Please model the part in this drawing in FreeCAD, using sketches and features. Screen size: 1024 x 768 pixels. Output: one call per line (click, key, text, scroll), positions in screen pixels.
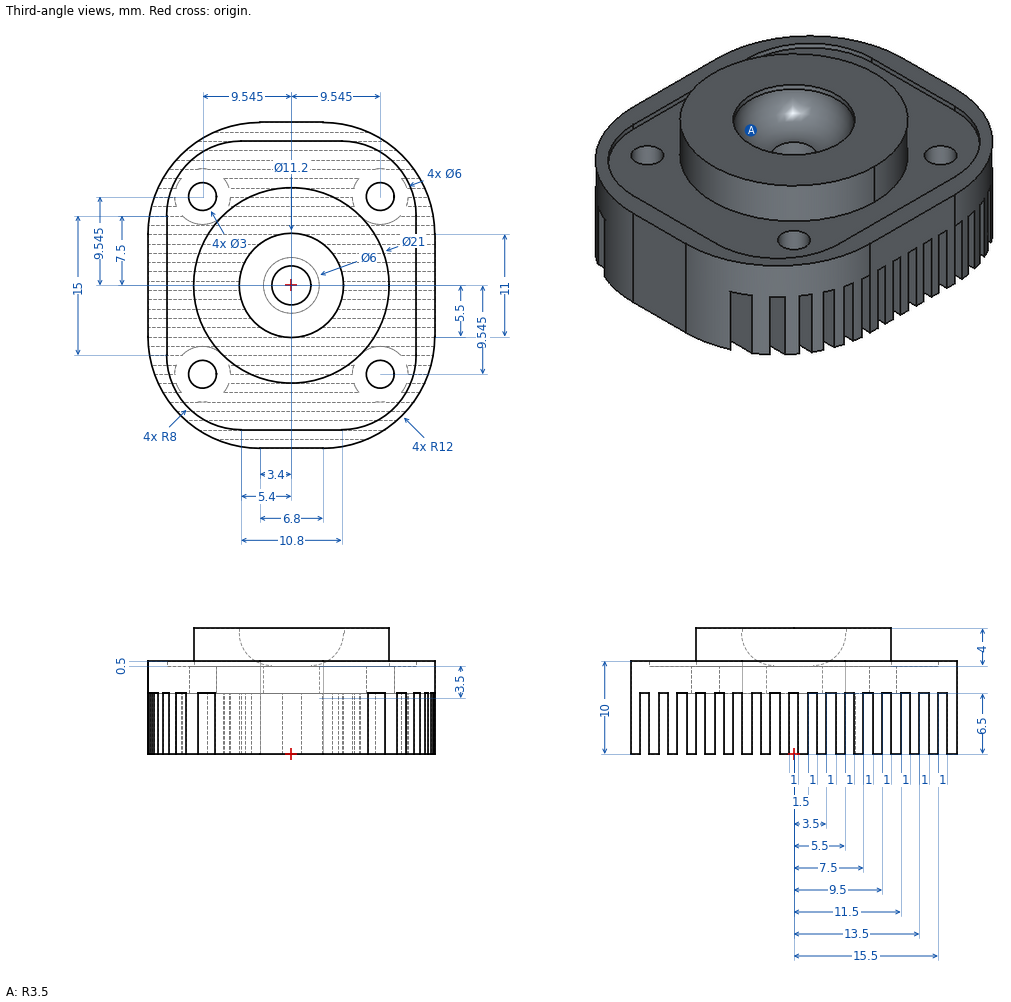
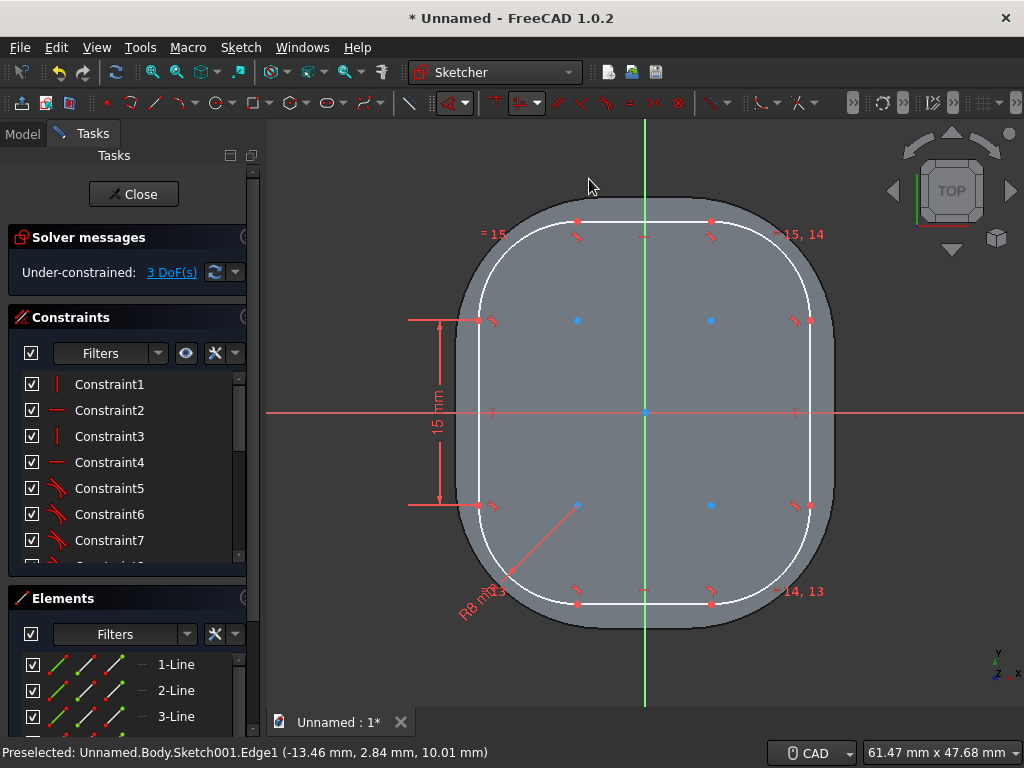
click(618, 604)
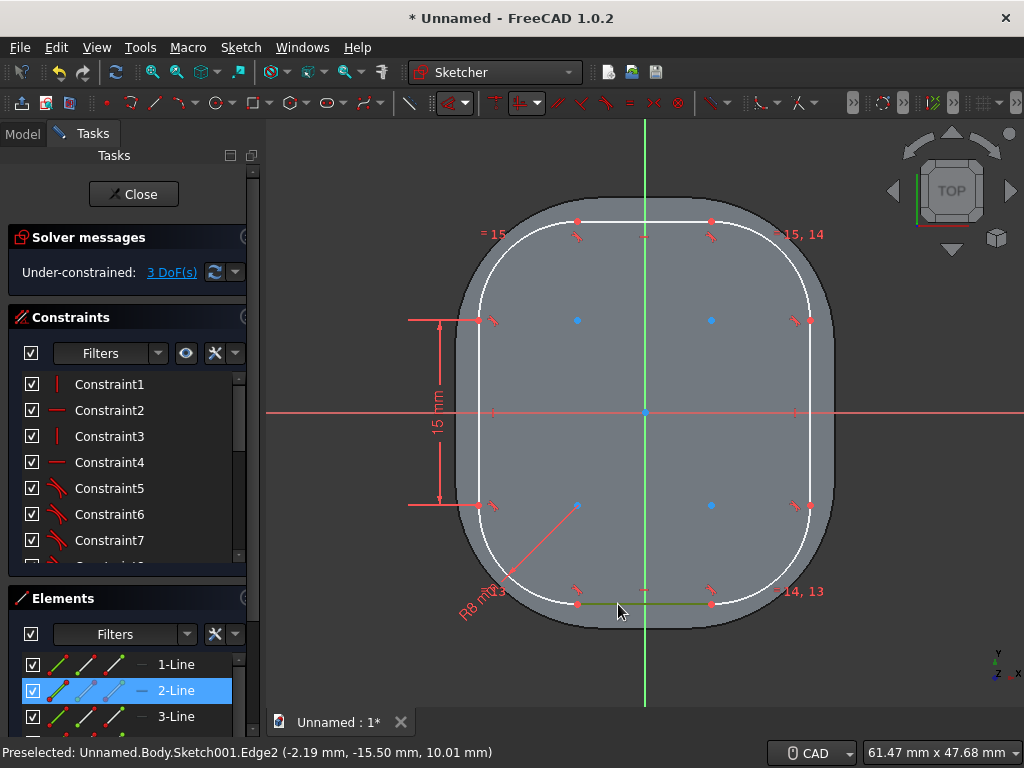
key(l)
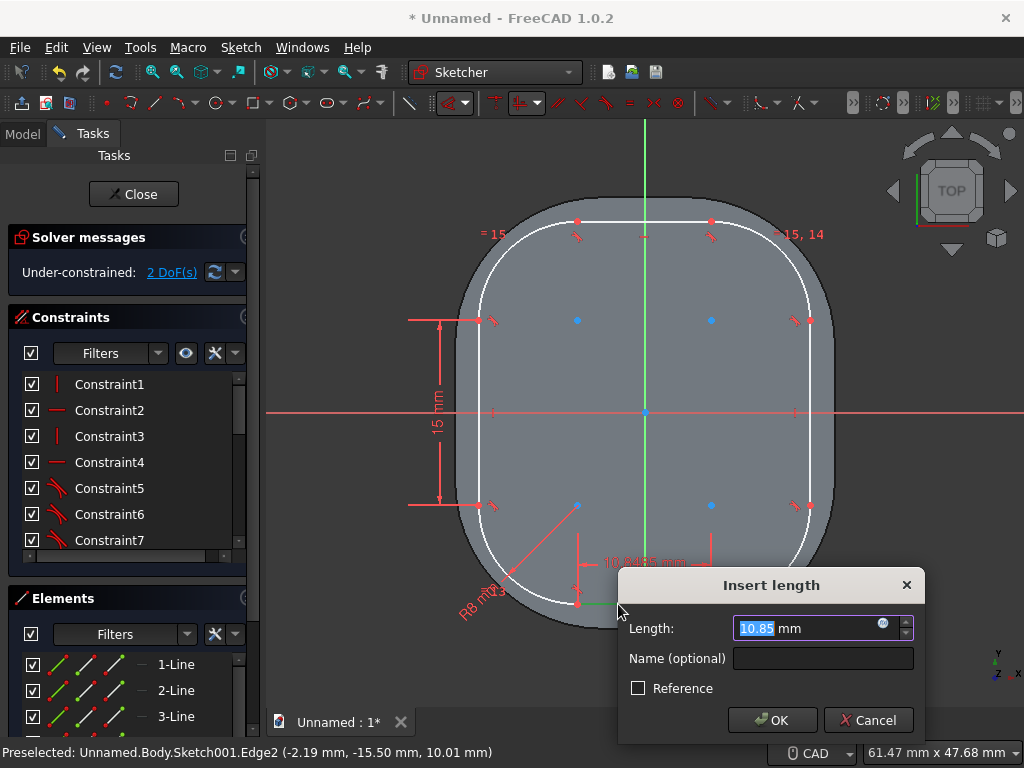
text(10.8)
key(Return)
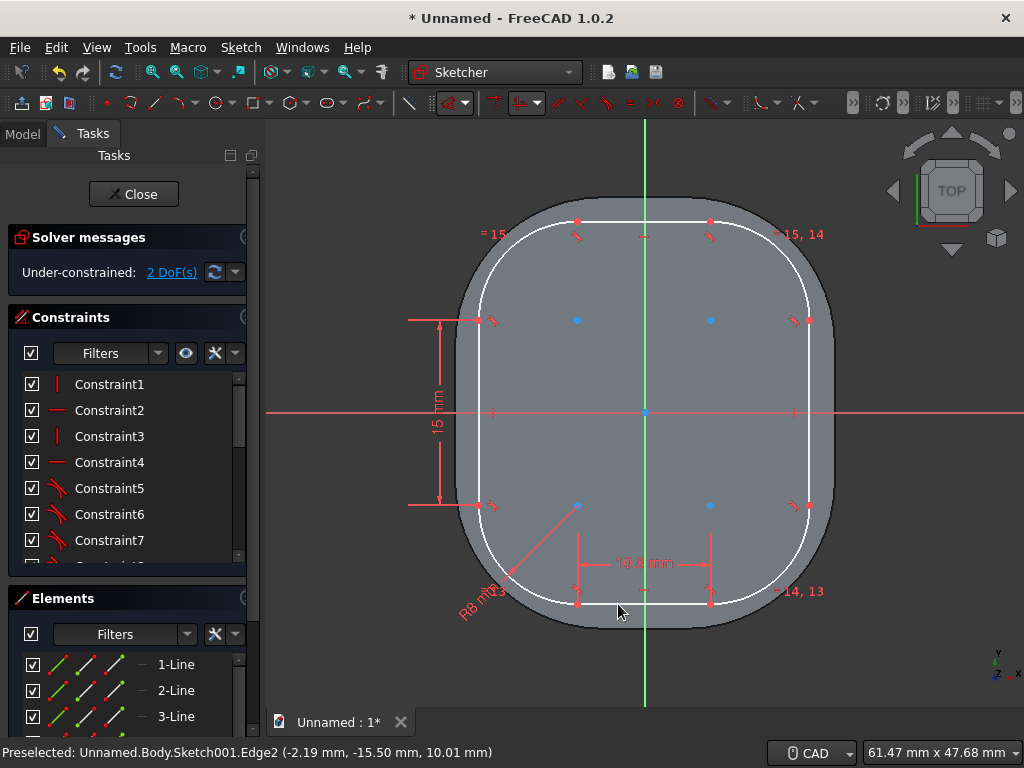
click(479, 320)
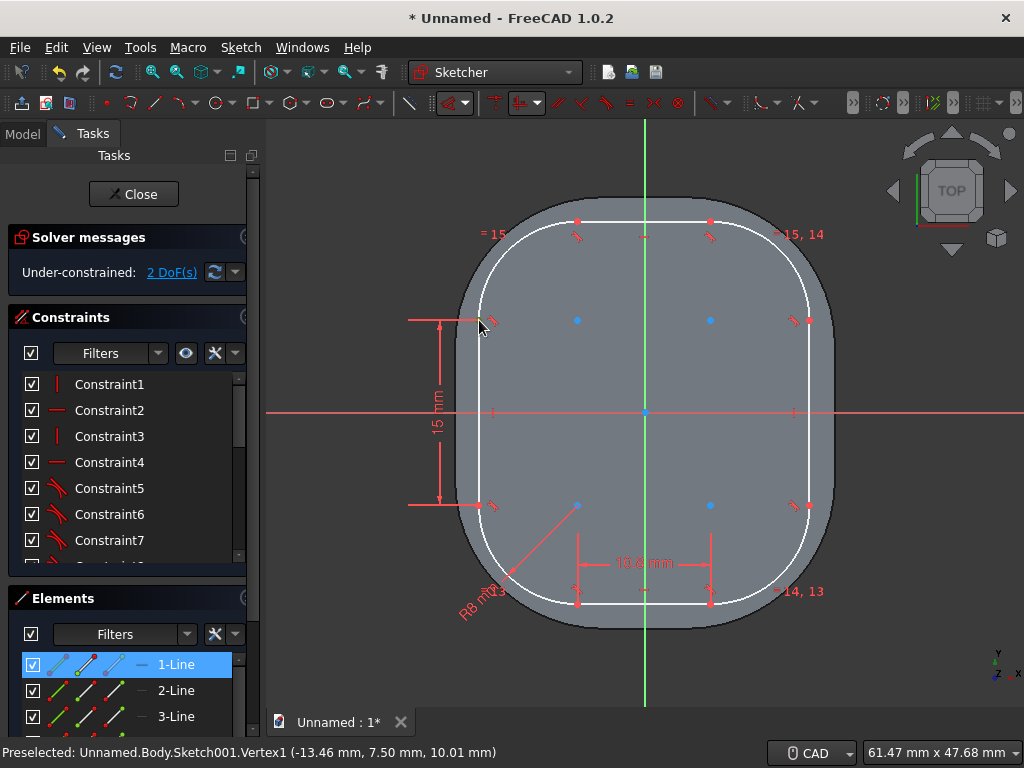
click(468, 104)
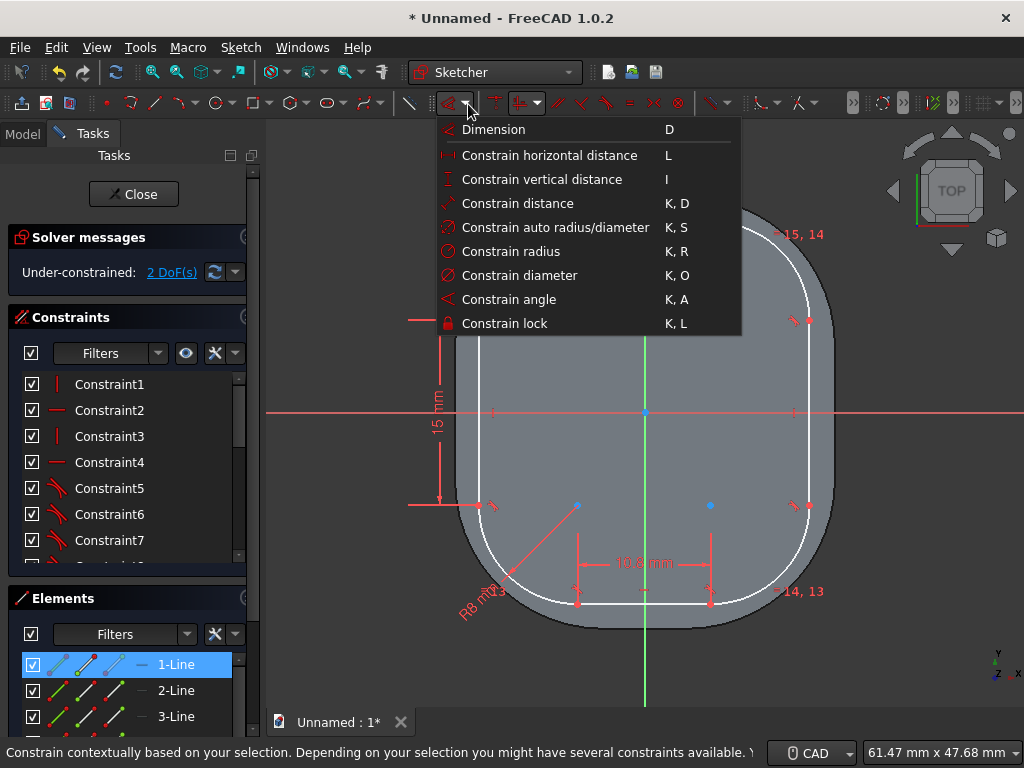
click(589, 179)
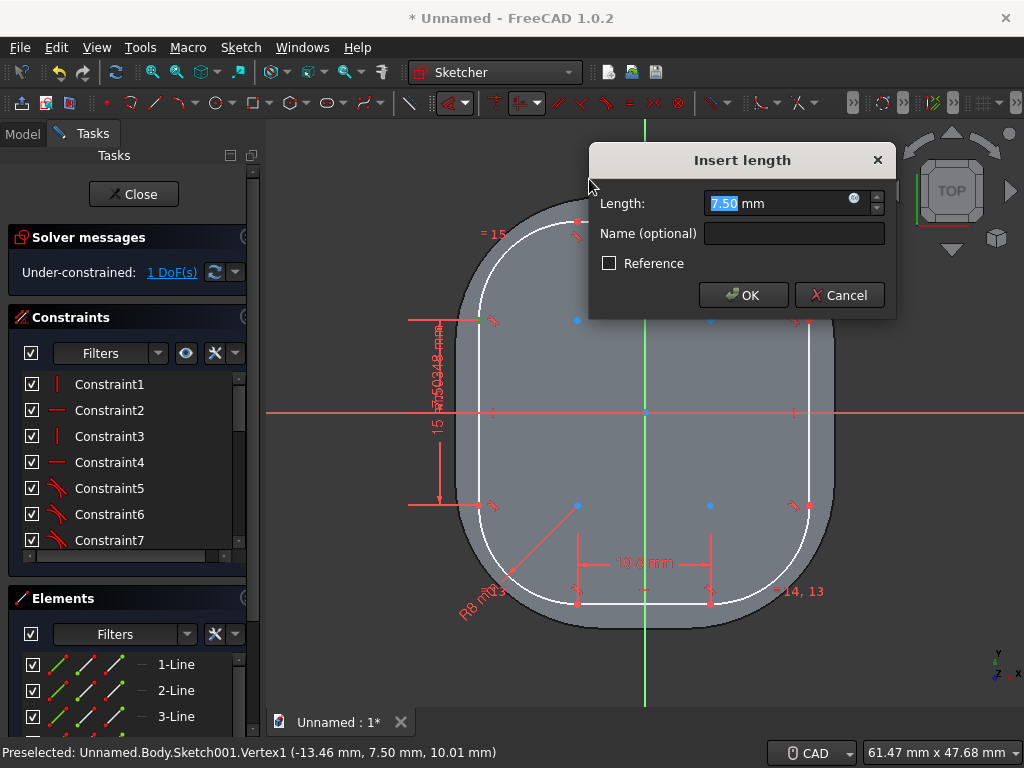
text(7.5)
key(Return)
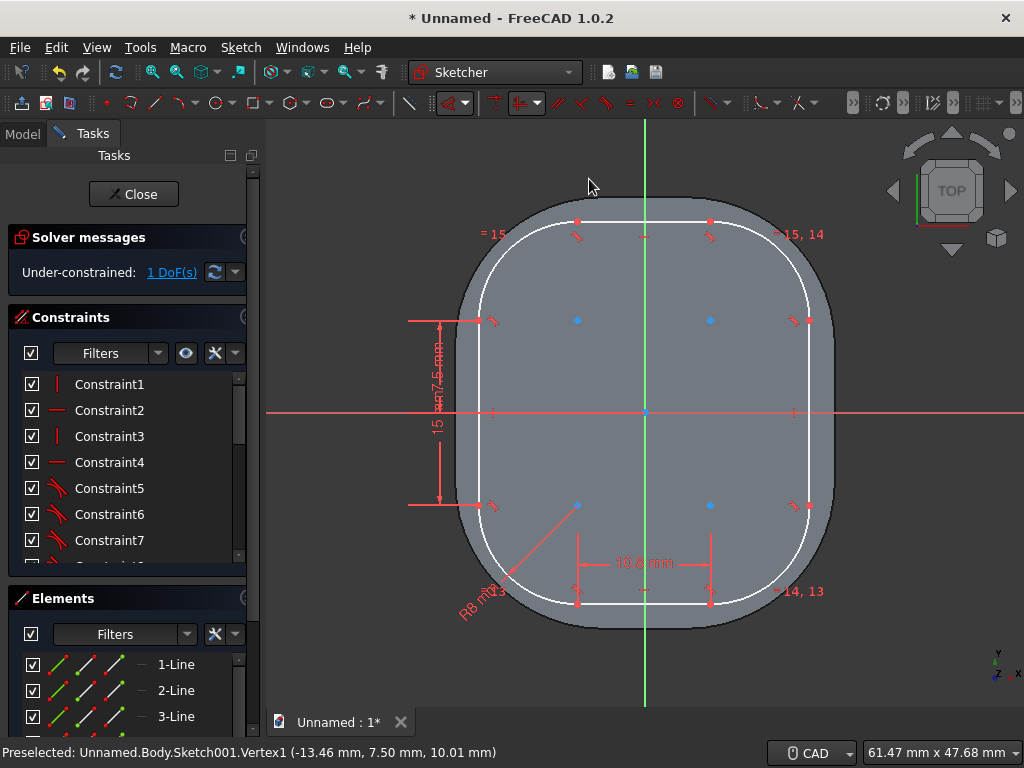
click(578, 604)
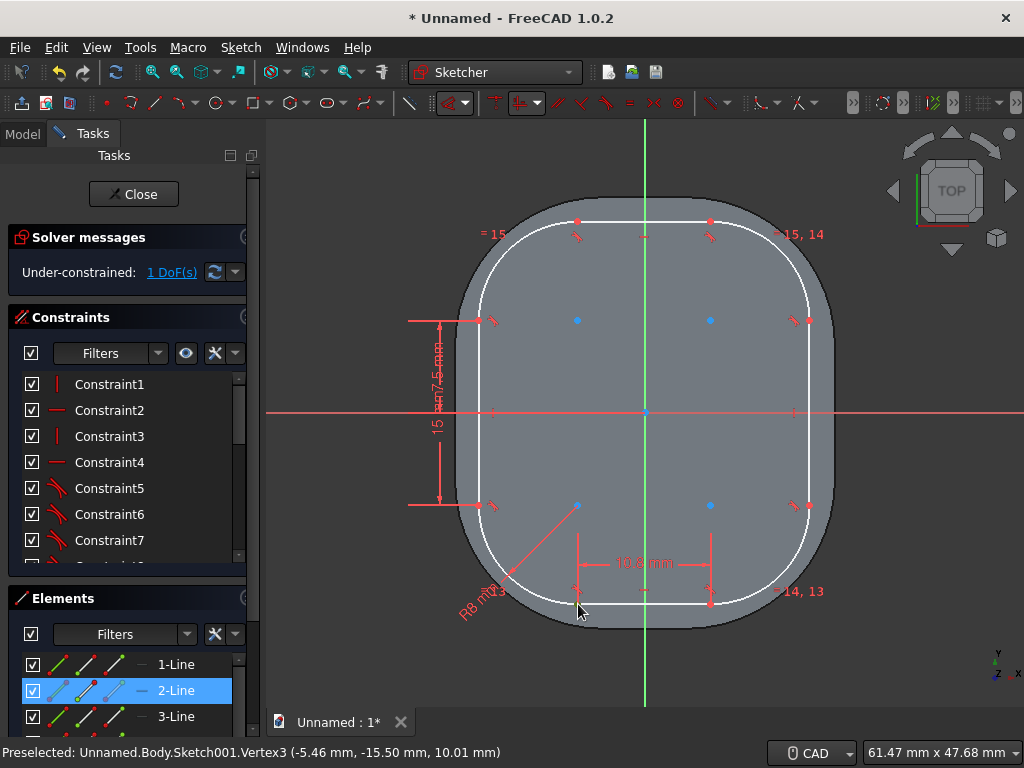
key(l)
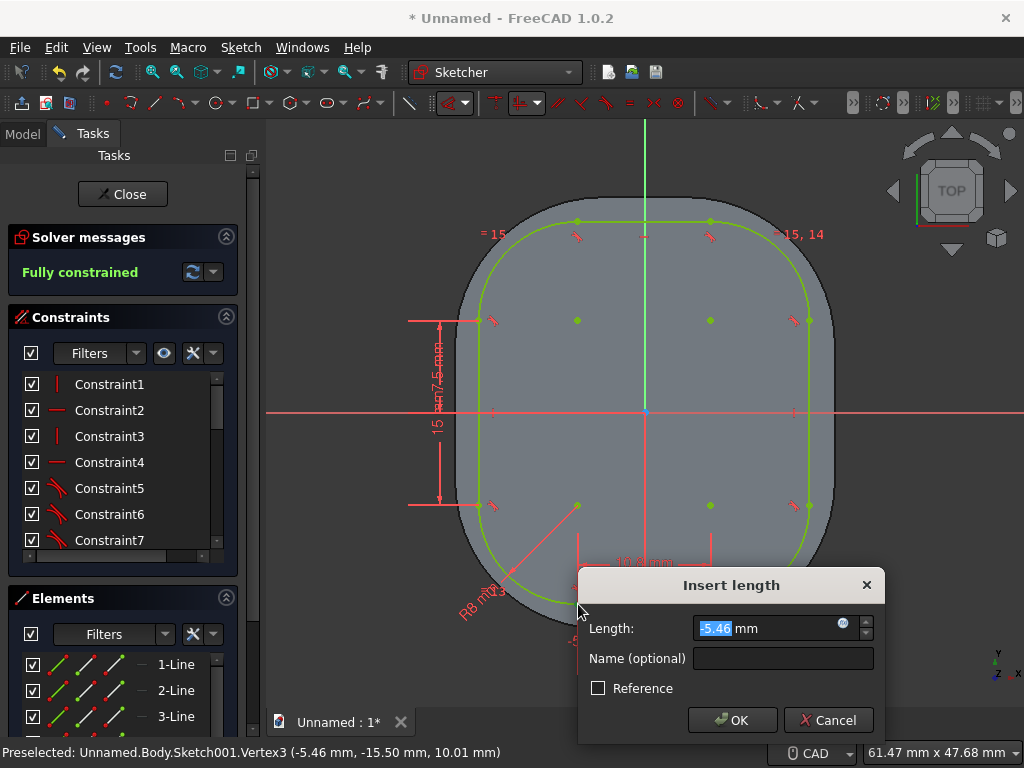
text(-5.4)
key(Return)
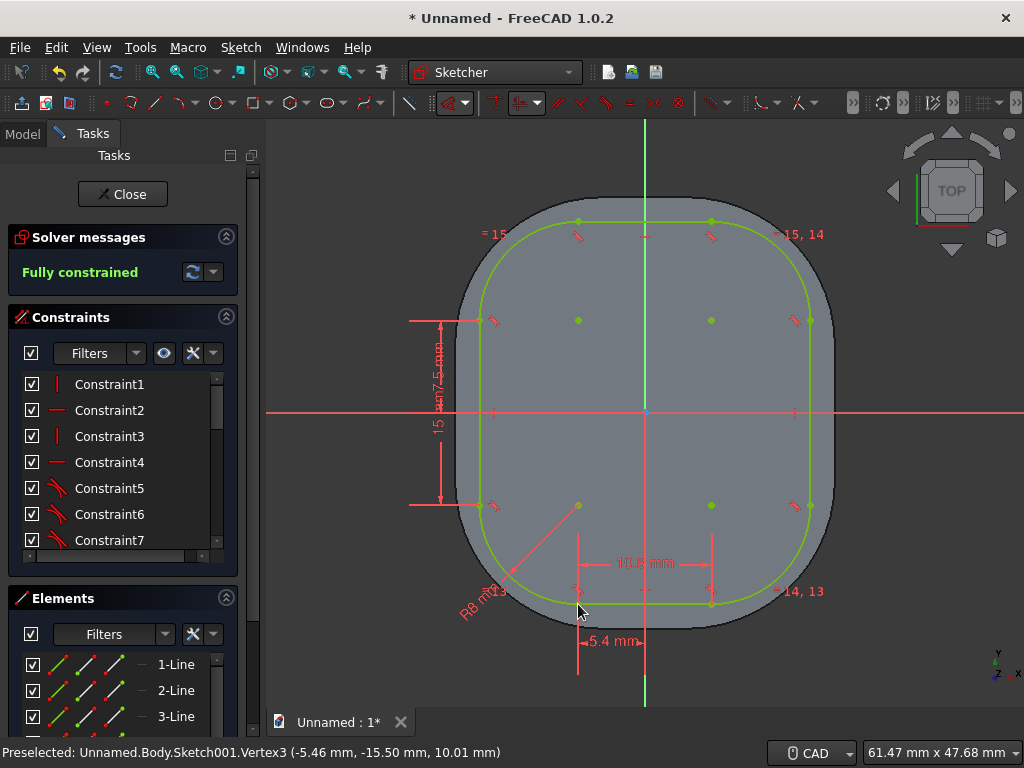
click(123, 194)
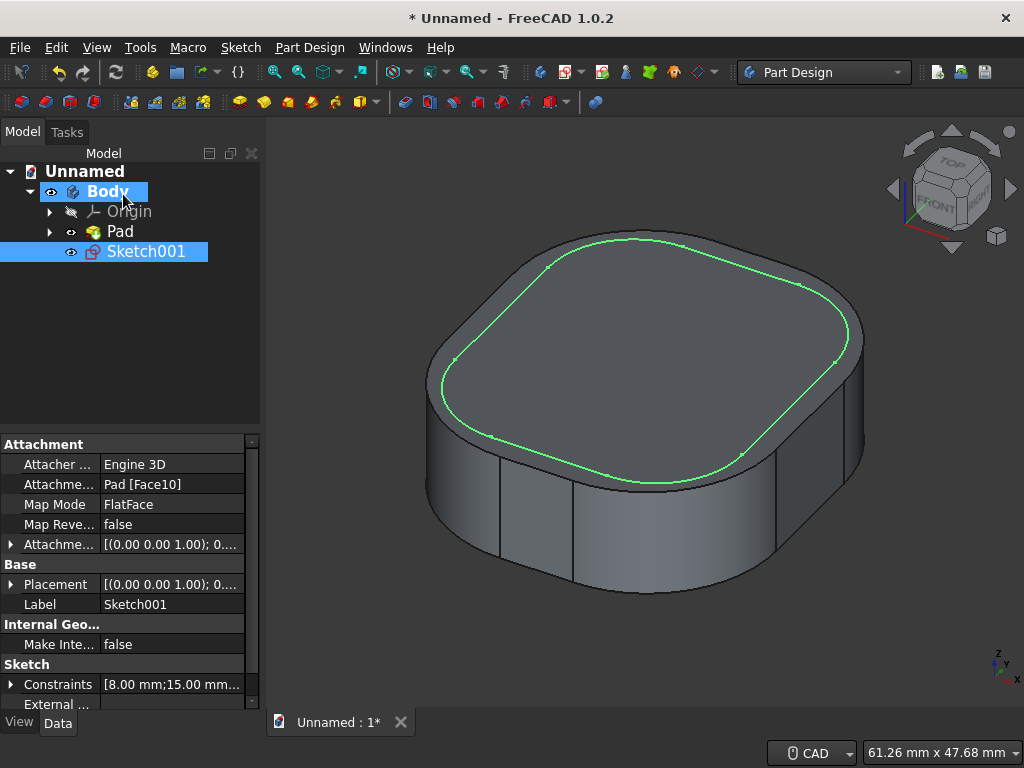
click(406, 102)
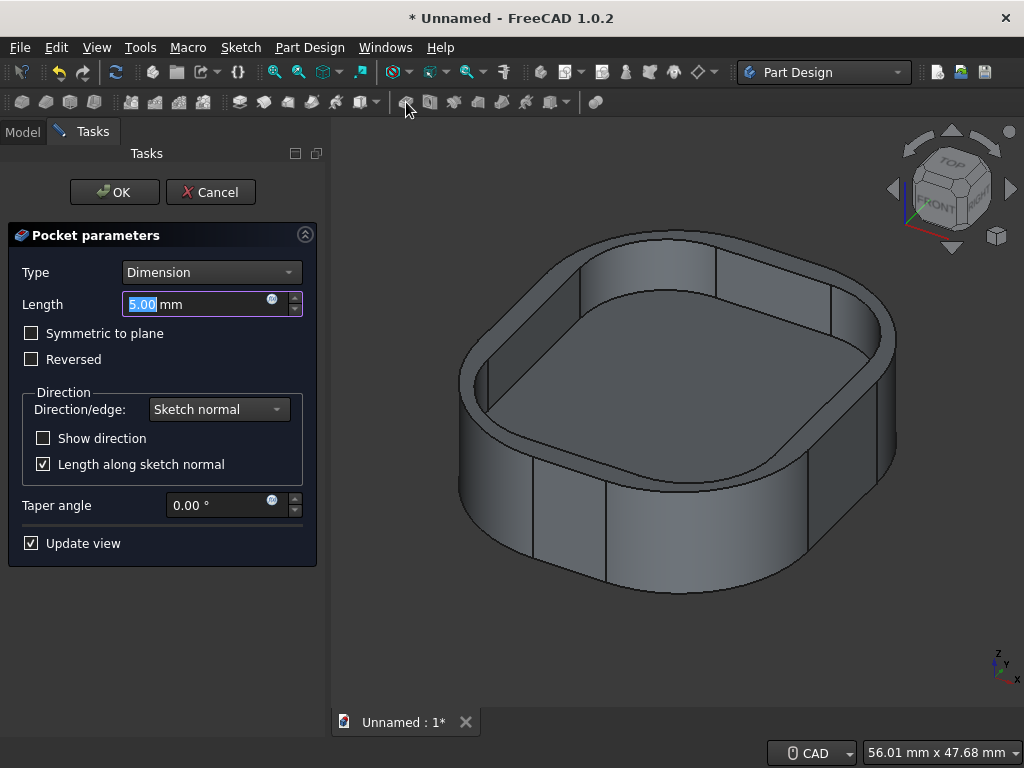
text(0.5)
key(Tab)